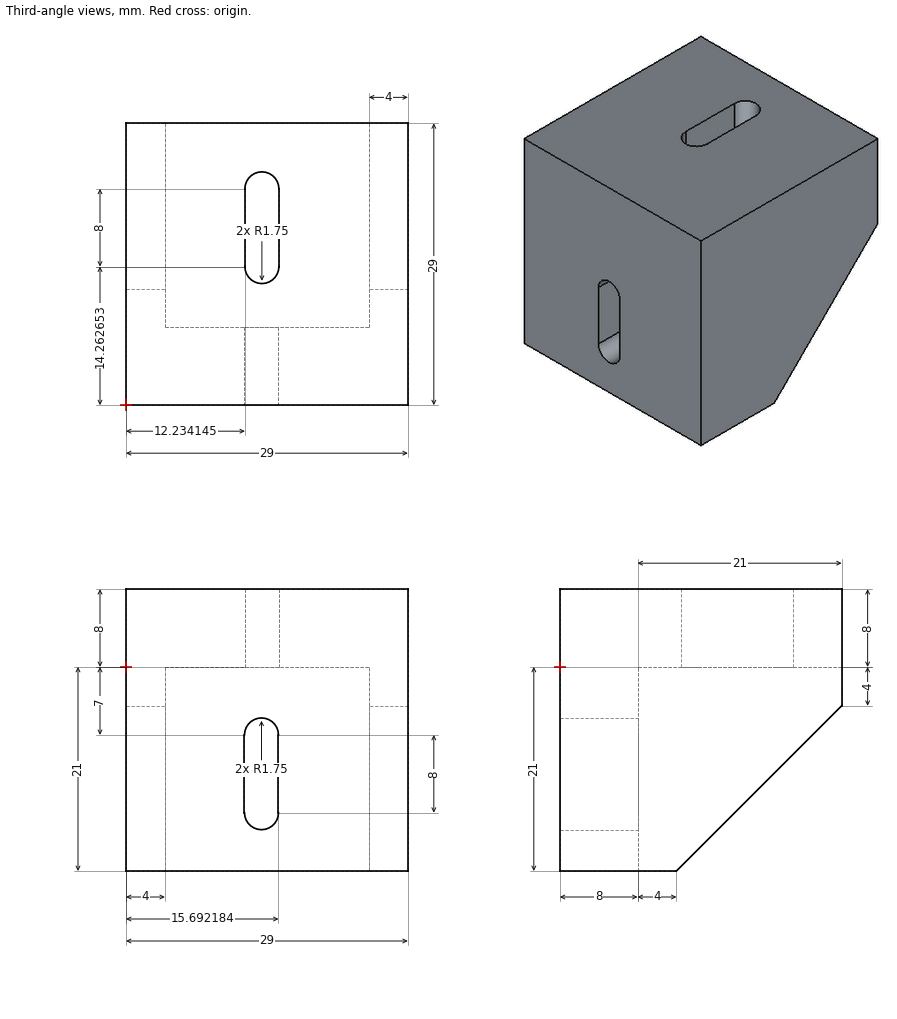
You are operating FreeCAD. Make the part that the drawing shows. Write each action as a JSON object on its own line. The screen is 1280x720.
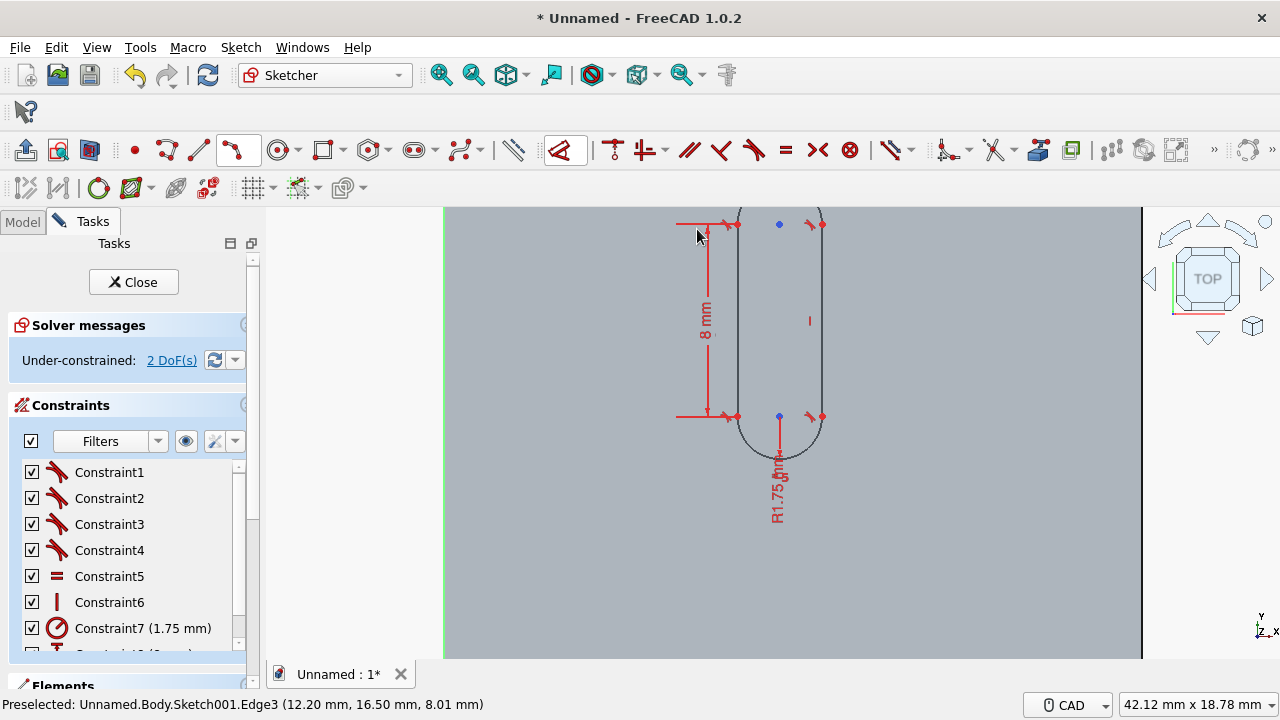
{"action": "left_click", "coordinate": [738, 417]}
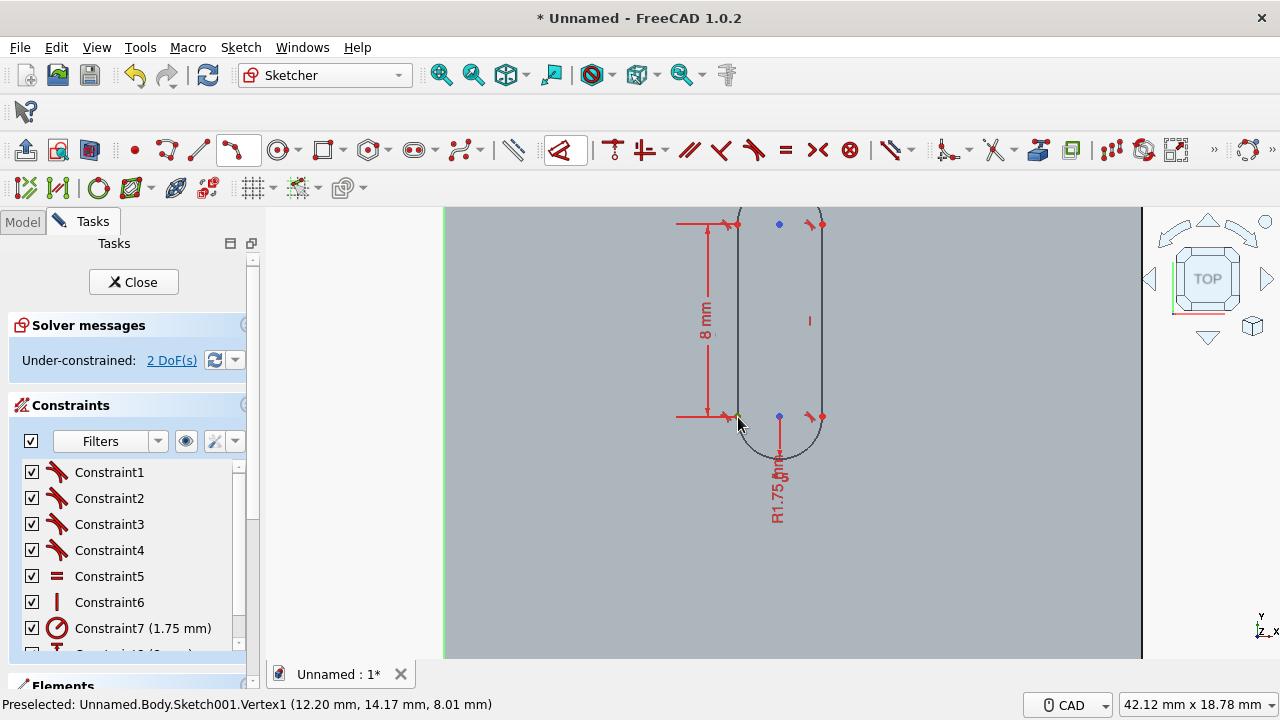
{"action": "key", "text": "l"}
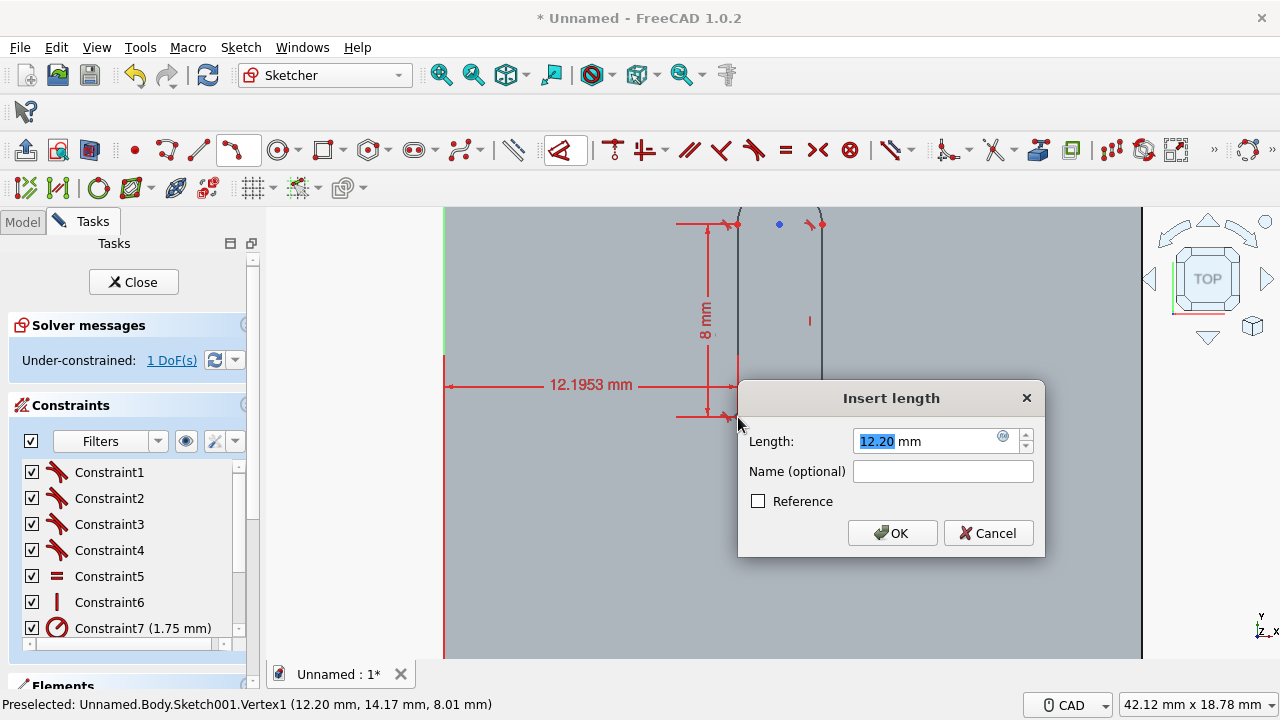
{"action": "type", "text": "12.234145"}
{"action": "key", "text": "Return"}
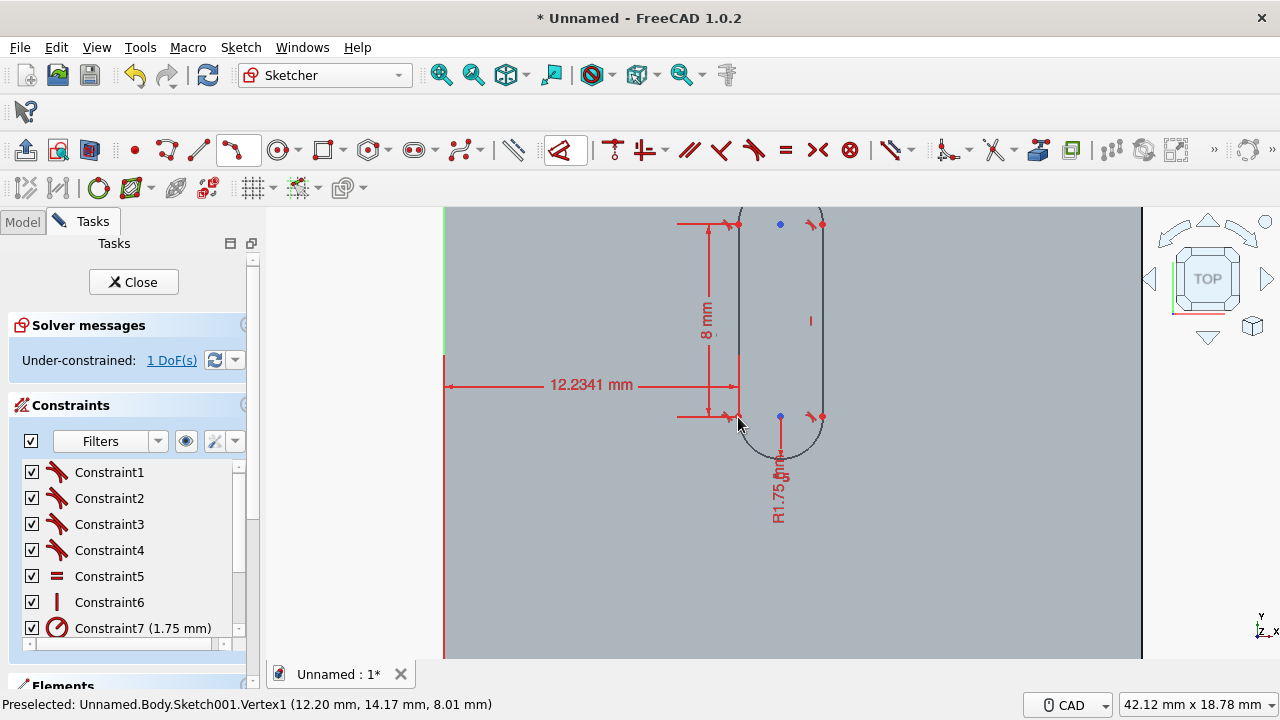
{"action": "left_click", "coordinate": [739, 417]}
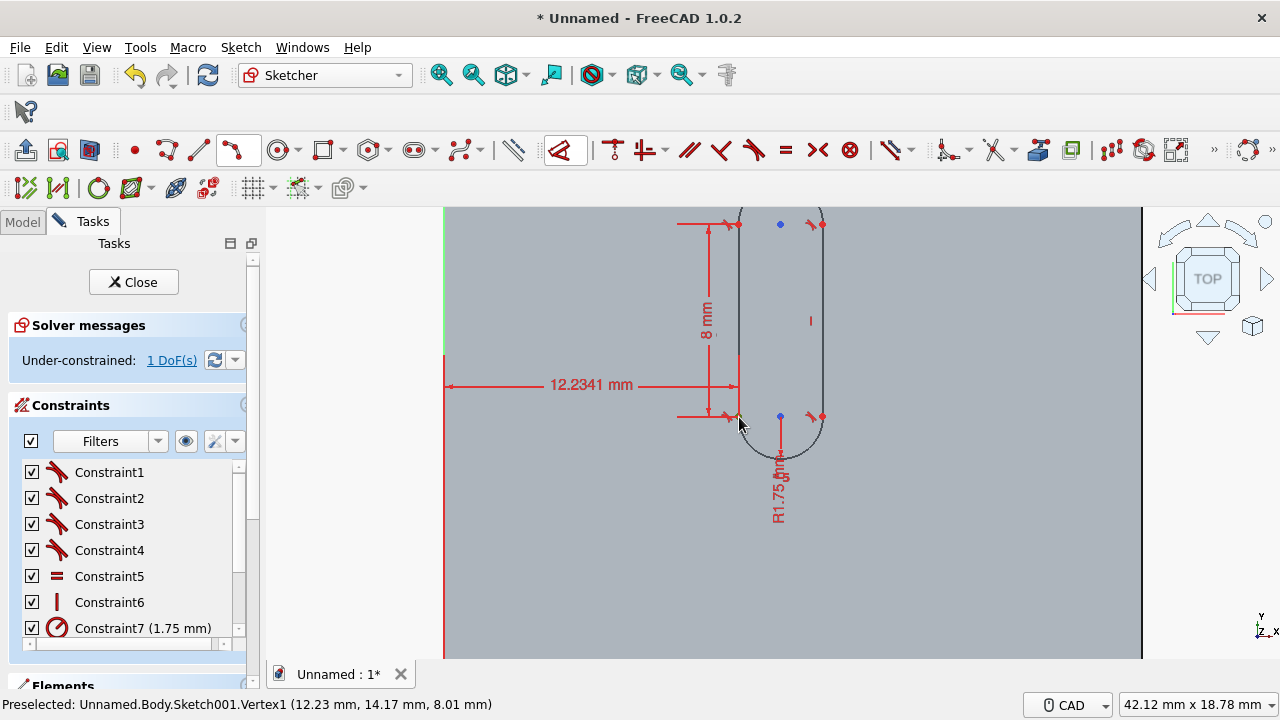
{"action": "key", "text": "i"}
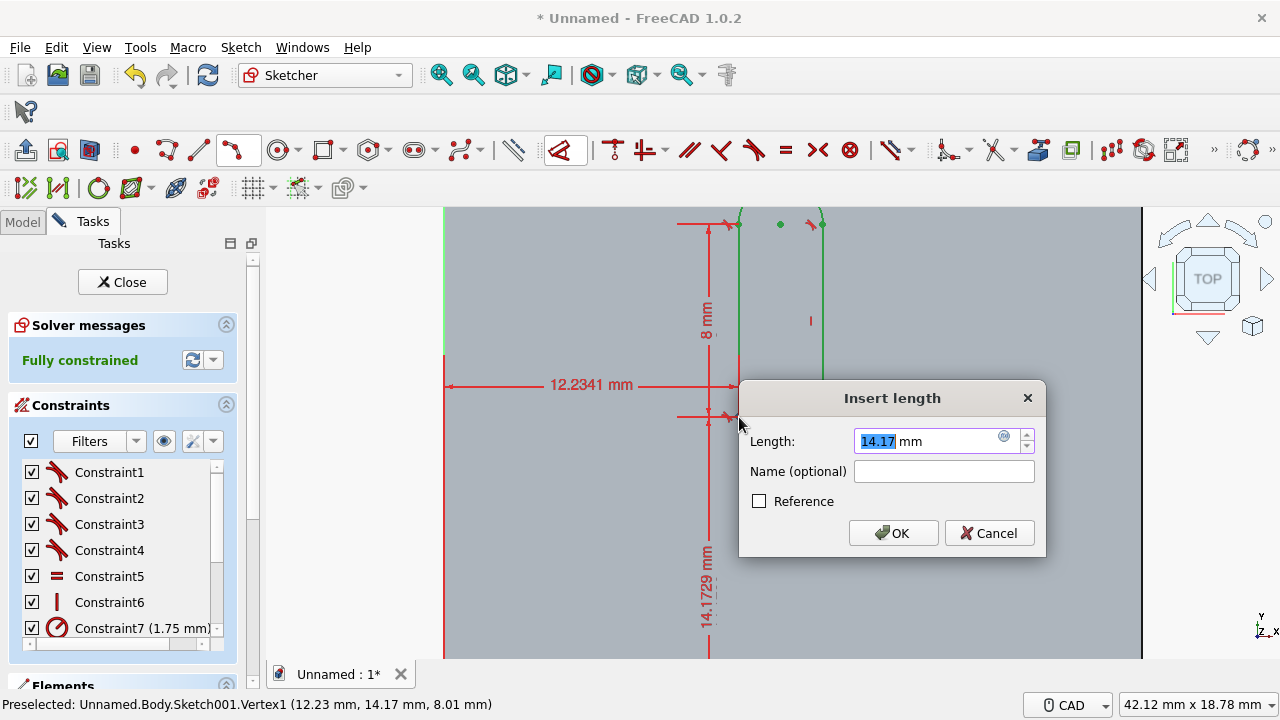
{"action": "type", "text": "14.262653"}
{"action": "key", "text": "Return"}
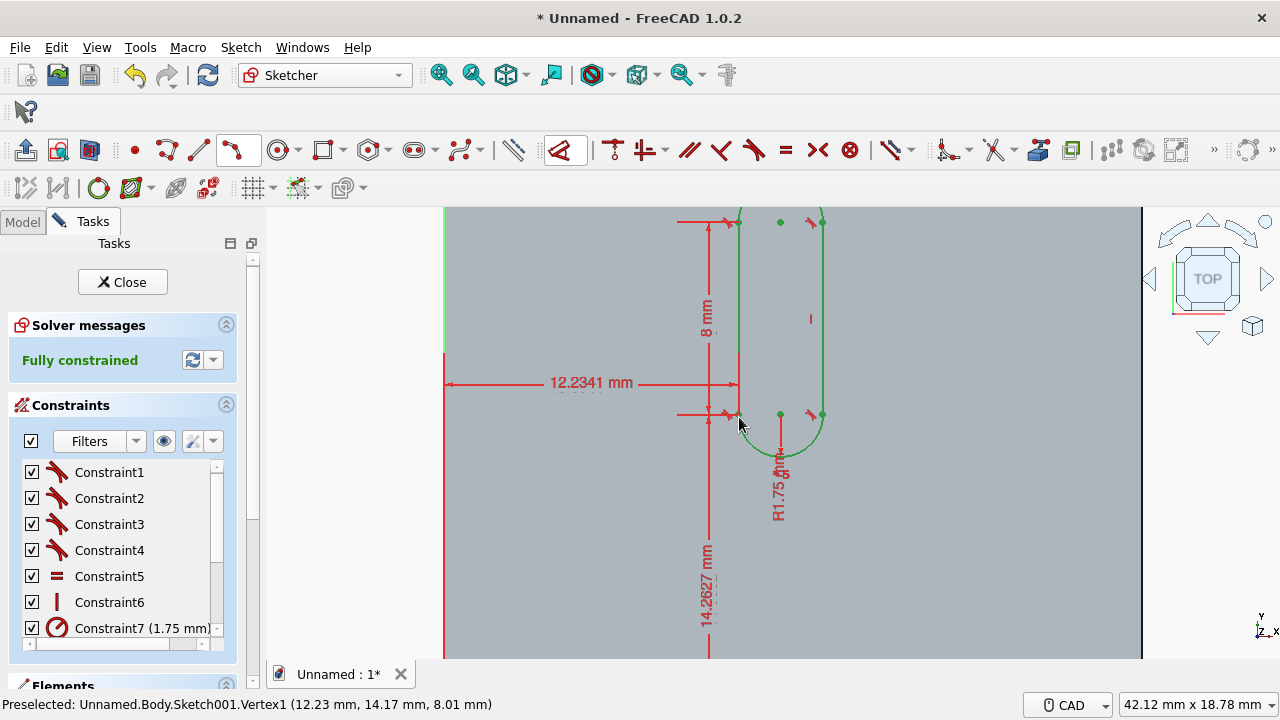
{"action": "left_click", "coordinate": [123, 282]}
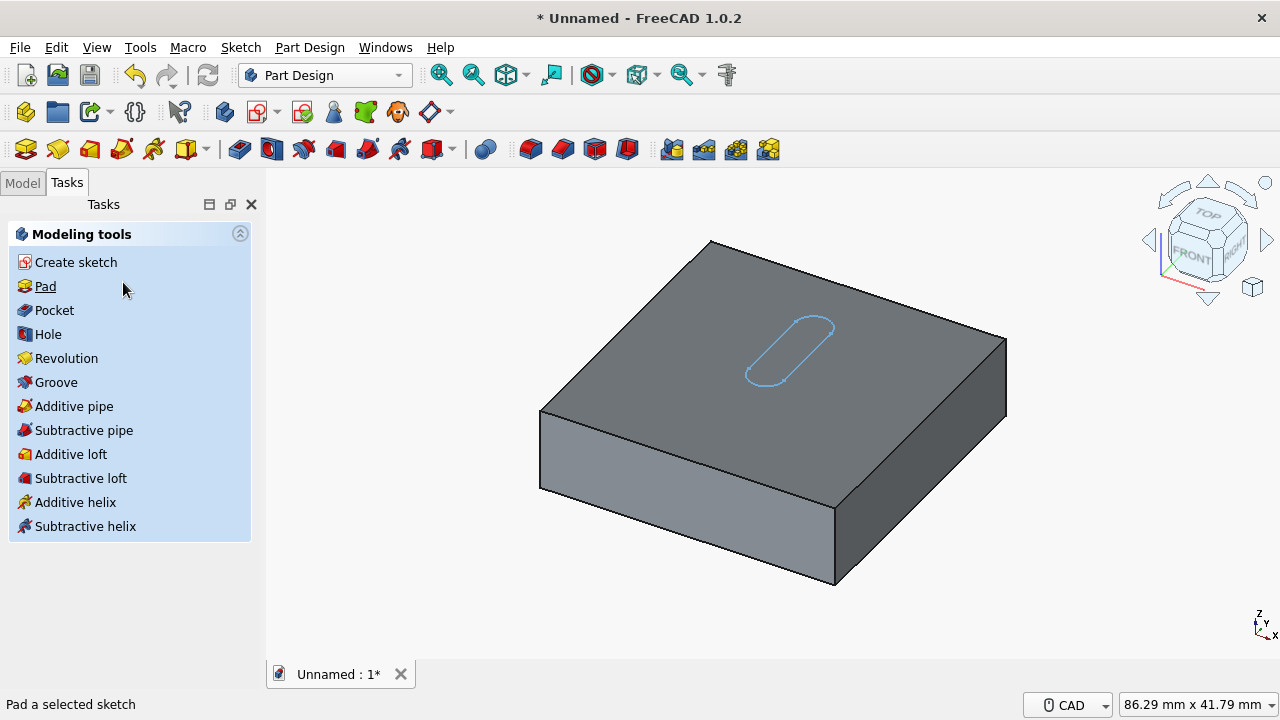
{"action": "left_click", "coordinate": [240, 150]}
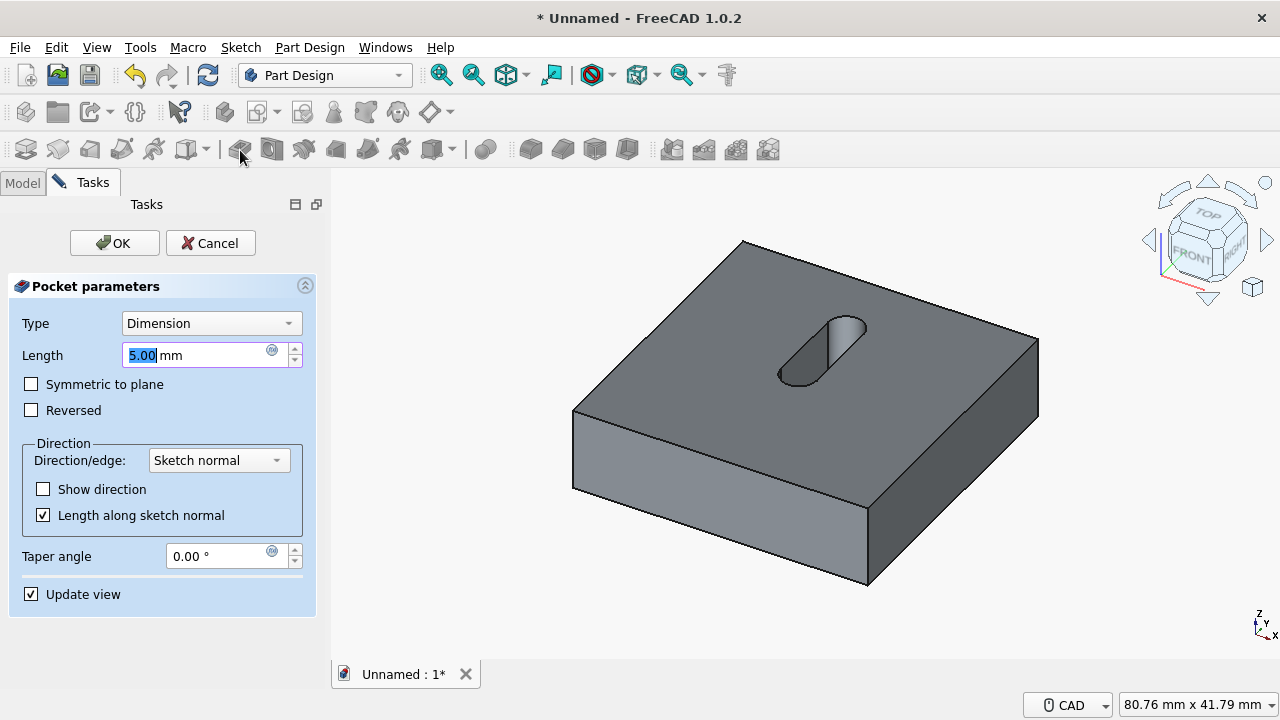
{"action": "type", "text": "8"}
{"action": "key", "text": "Tab"}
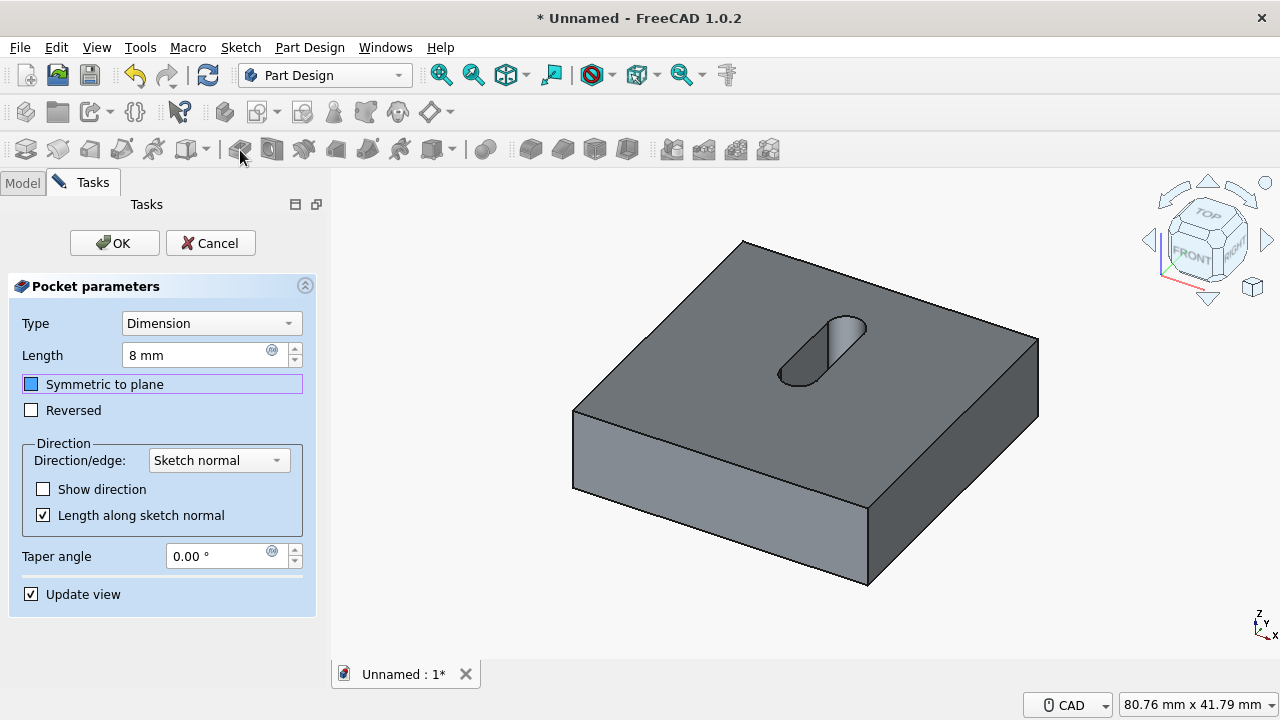
{"action": "left_click", "coordinate": [115, 243]}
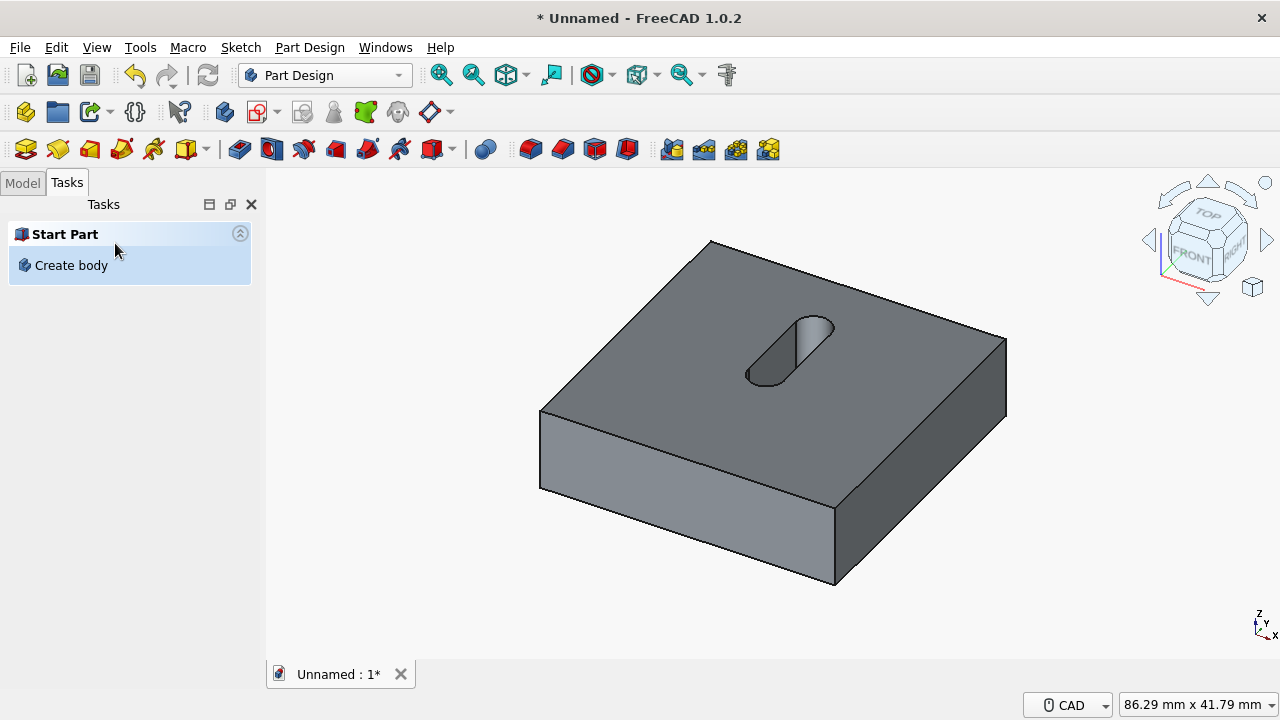
{"action": "left_click", "coordinate": [772, 525]}